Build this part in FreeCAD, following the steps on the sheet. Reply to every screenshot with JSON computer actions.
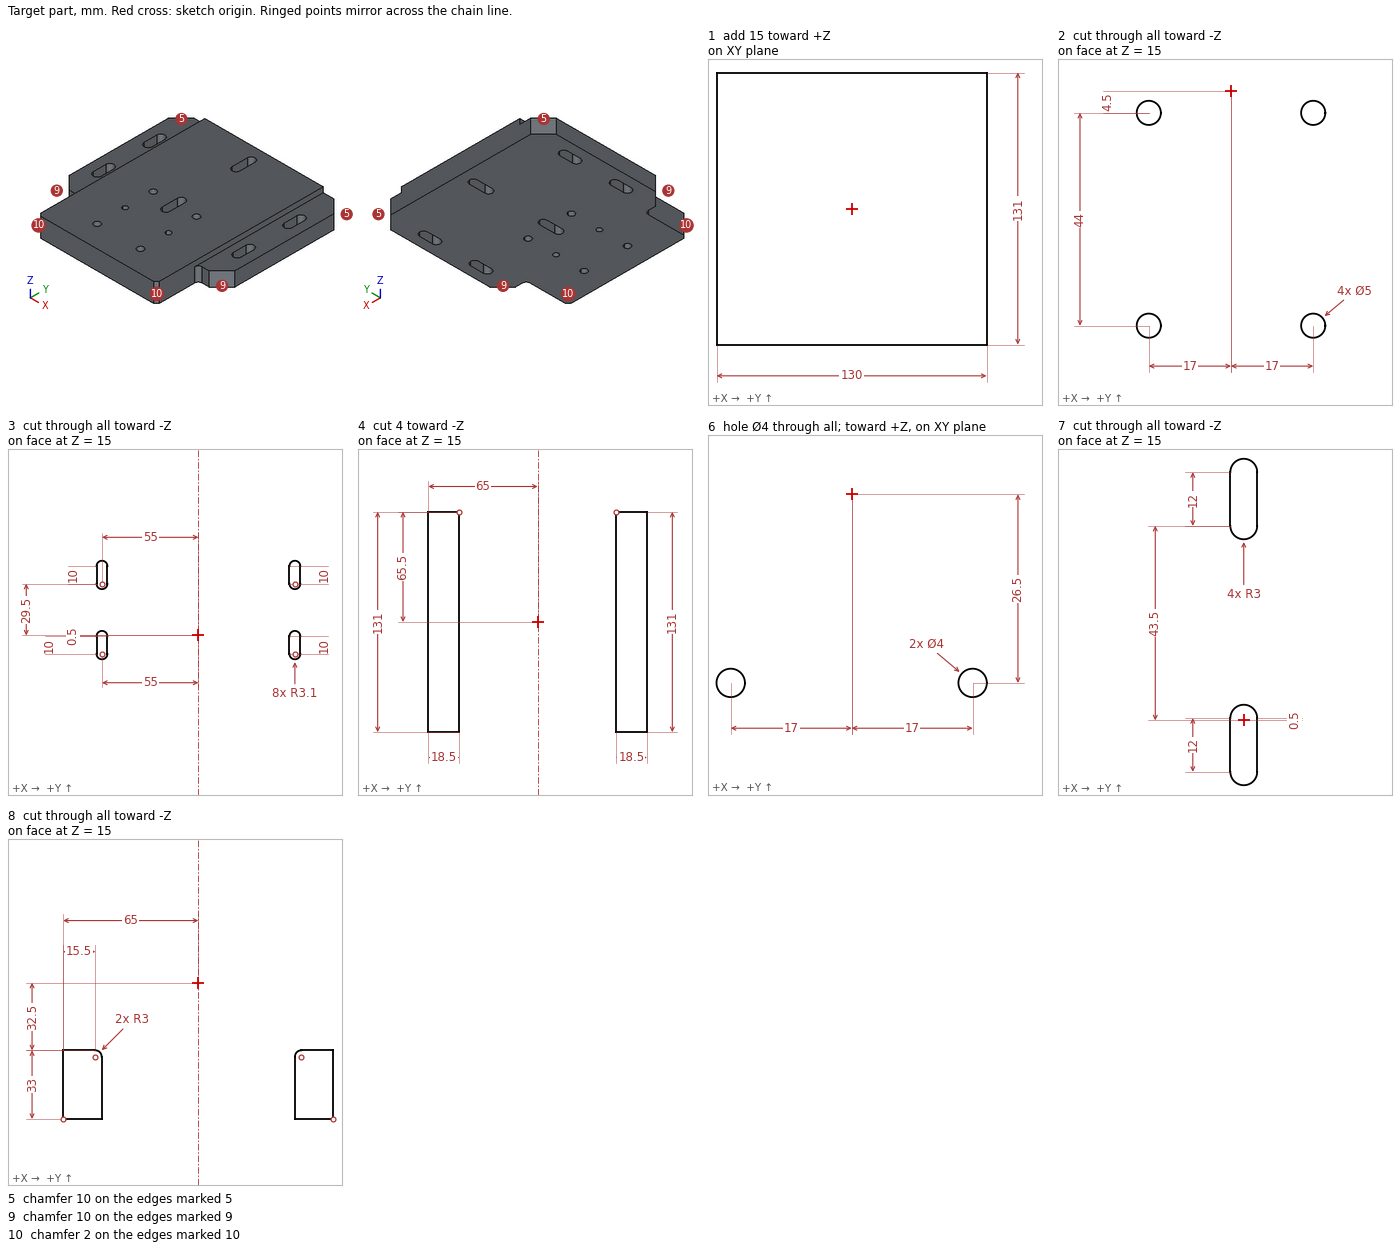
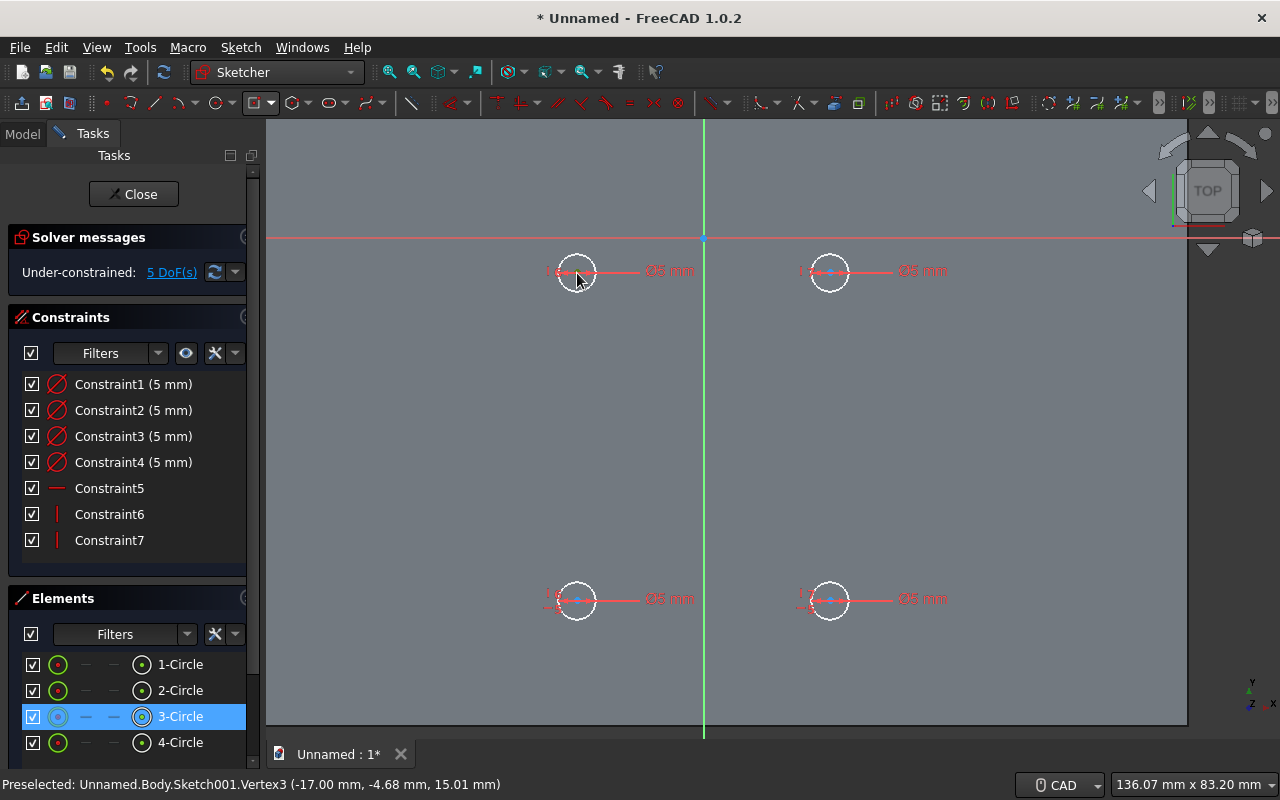
{"action": "left_click", "coordinate": [830, 273]}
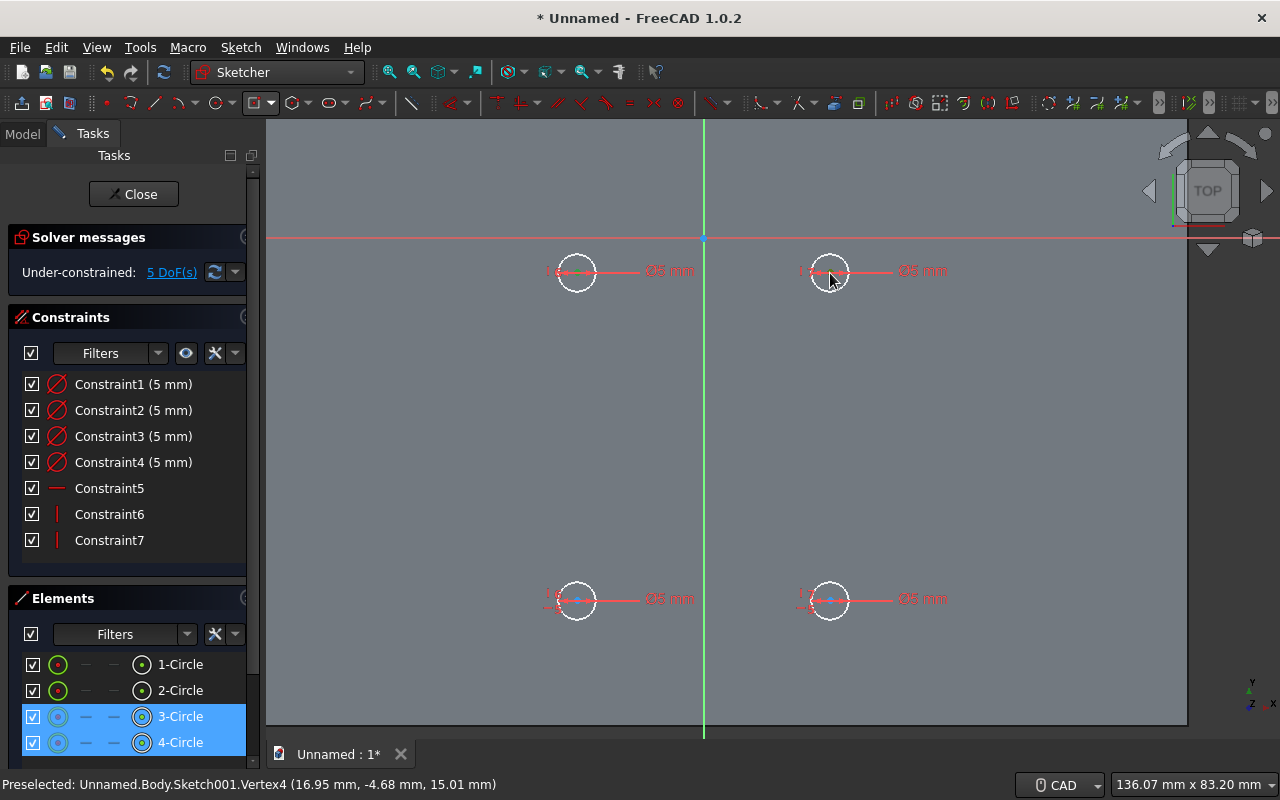
{"action": "key", "text": "h"}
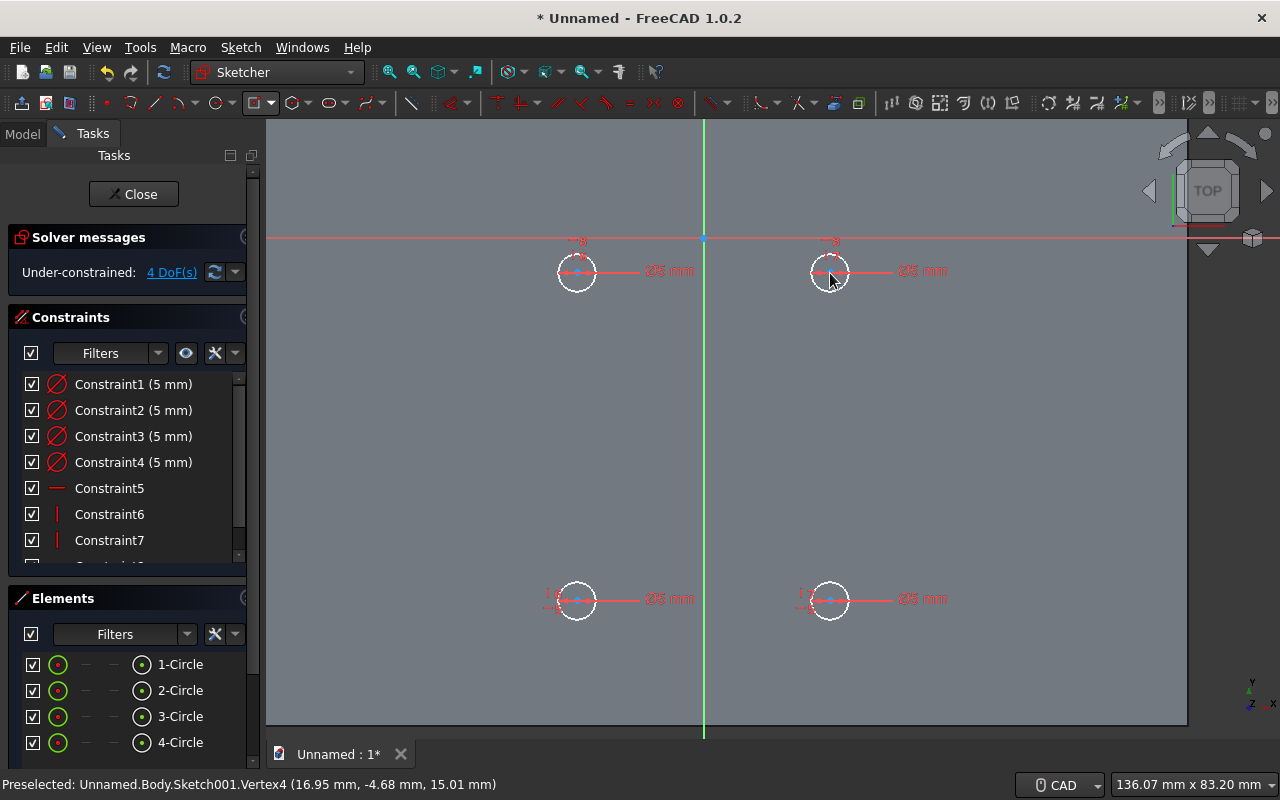
{"action": "left_click", "coordinate": [450, 104]}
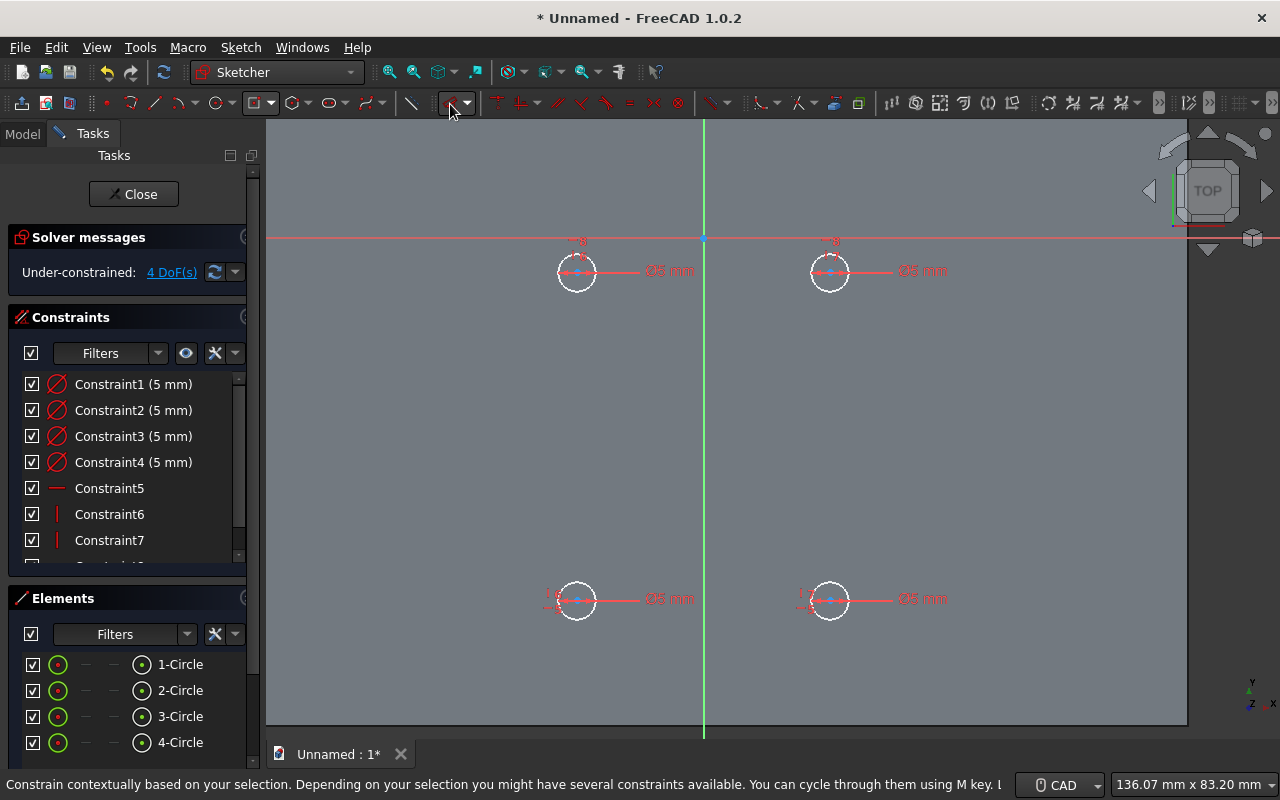
{"action": "left_click", "coordinate": [830, 601]}
{"action": "left_click", "coordinate": [767, 204]}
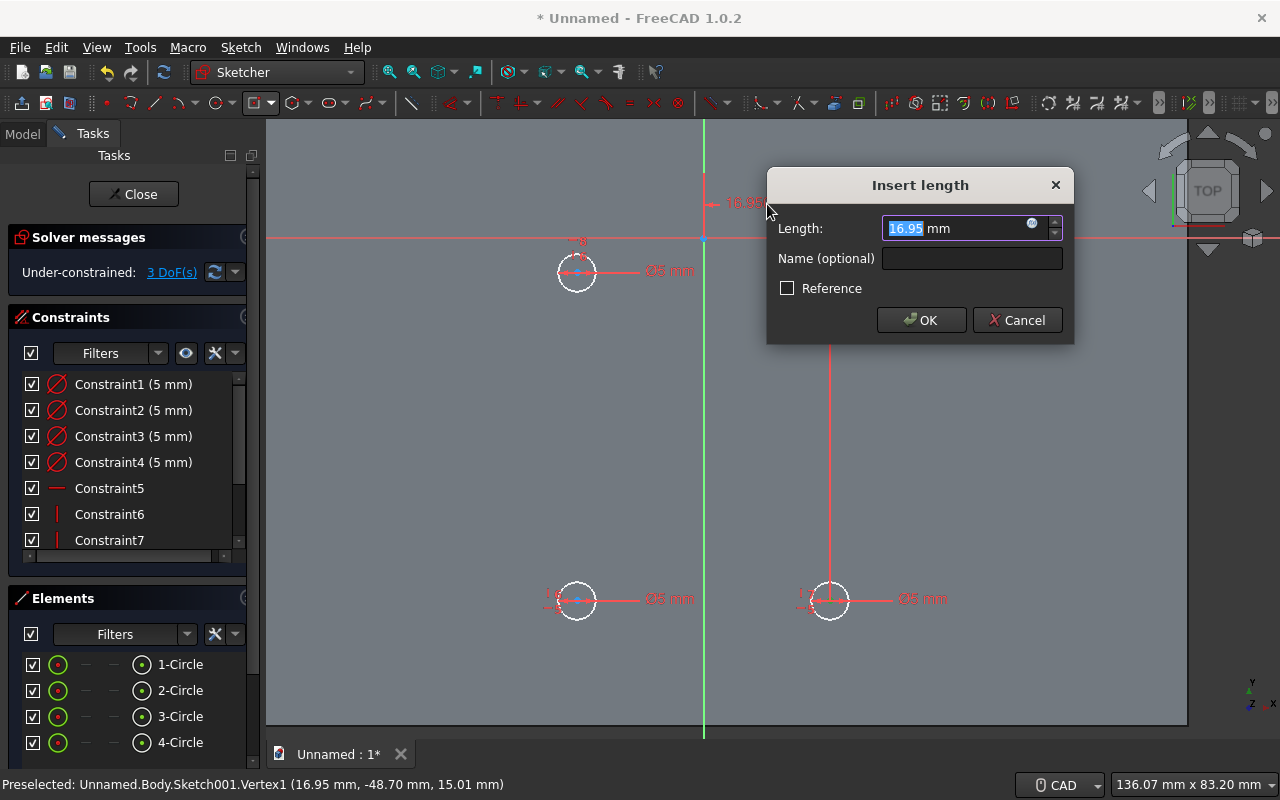
{"action": "type", "text": "17"}
{"action": "key", "text": "Return"}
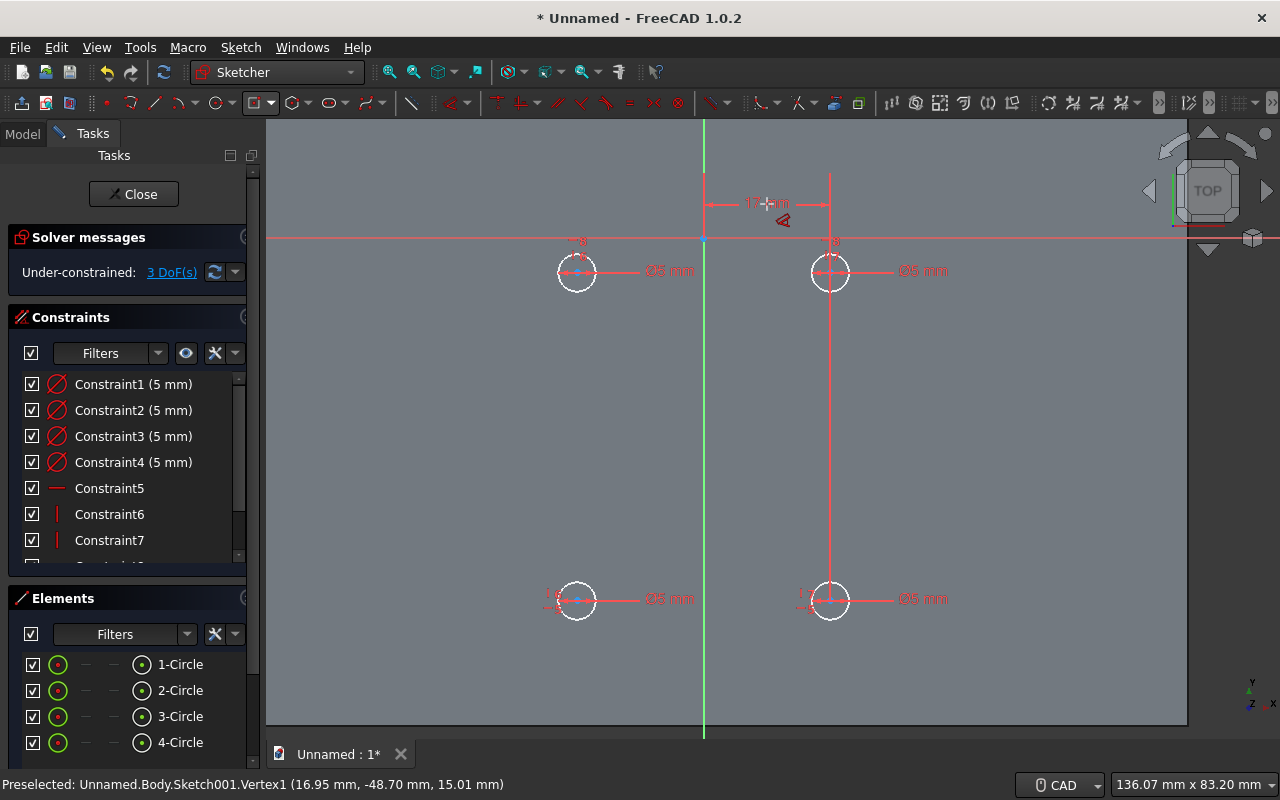
{"action": "left_click", "coordinate": [577, 601]}
{"action": "left_click", "coordinate": [640, 204]}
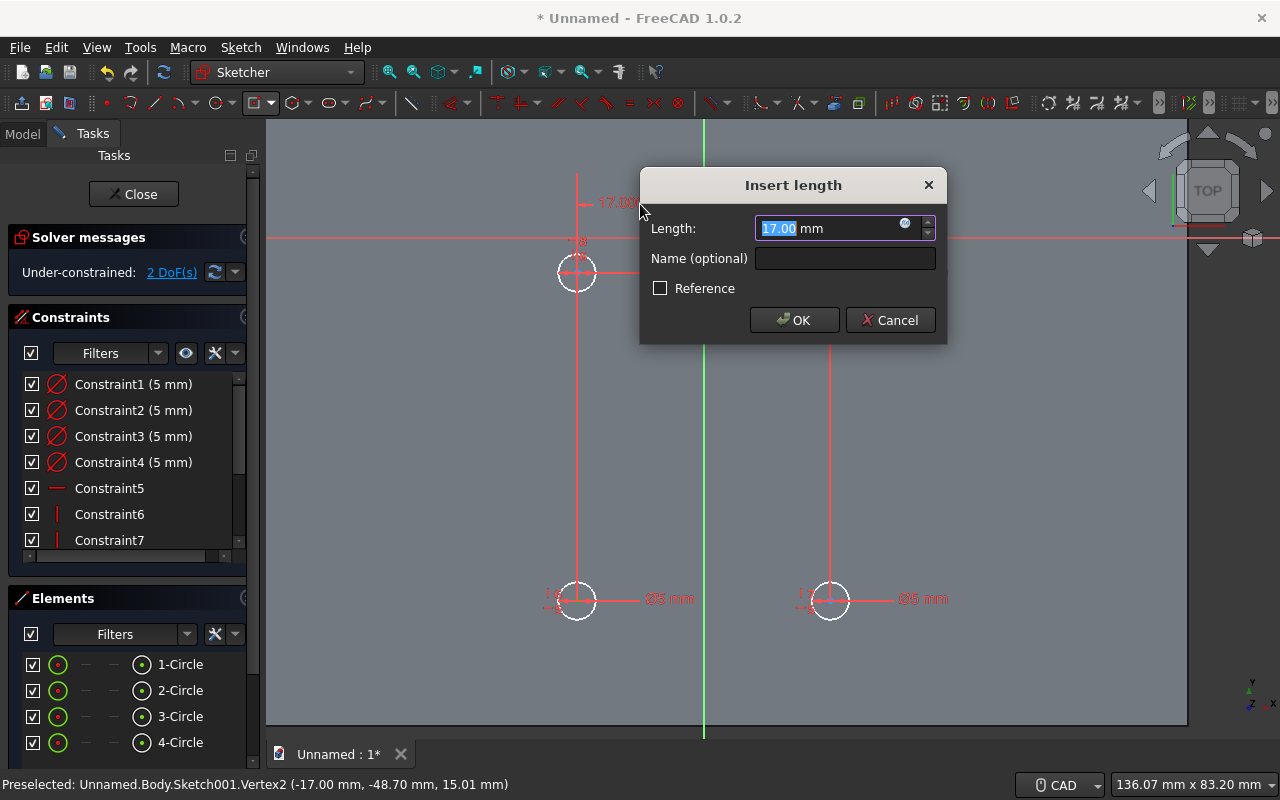
{"action": "type", "text": "17"}
{"action": "key", "text": "Return"}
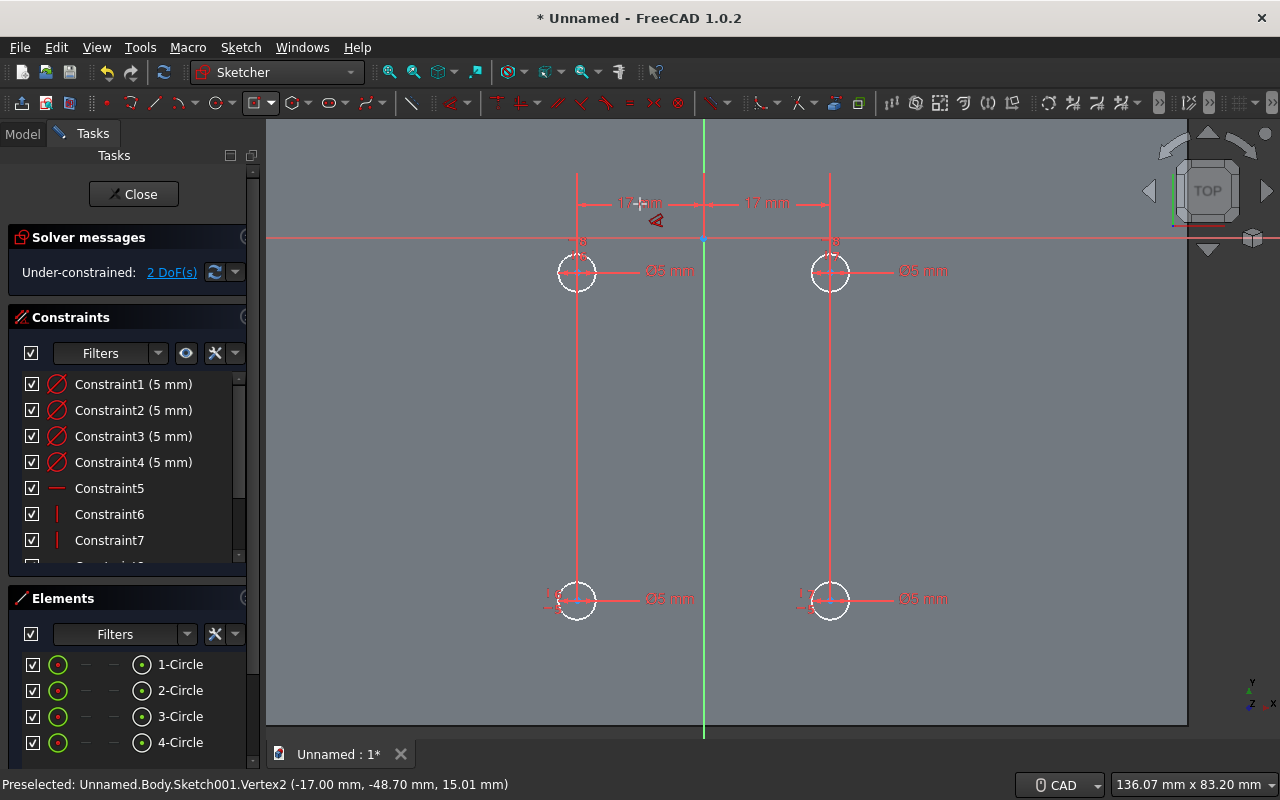
{"action": "left_click", "coordinate": [577, 273]}
{"action": "left_click", "coordinate": [543, 256]}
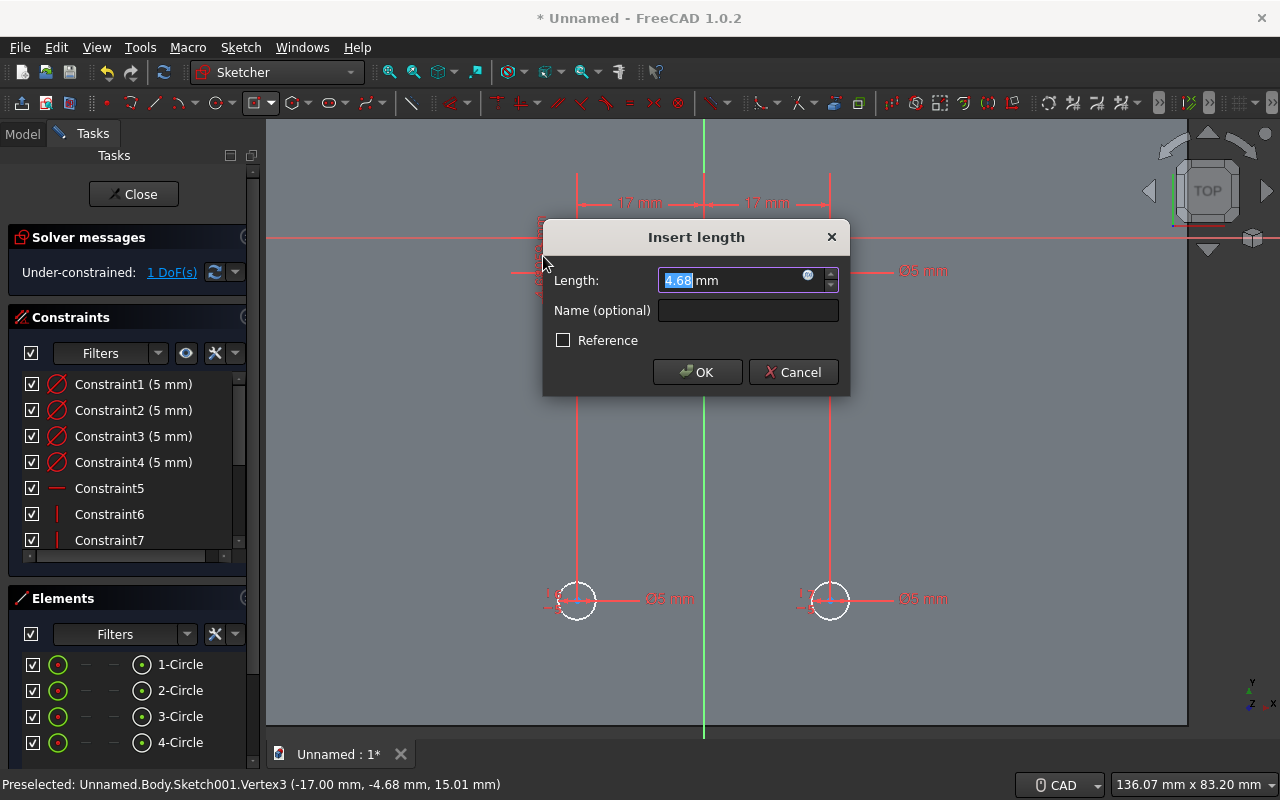
{"action": "type", "text": "4.5"}
{"action": "key", "text": "Return"}